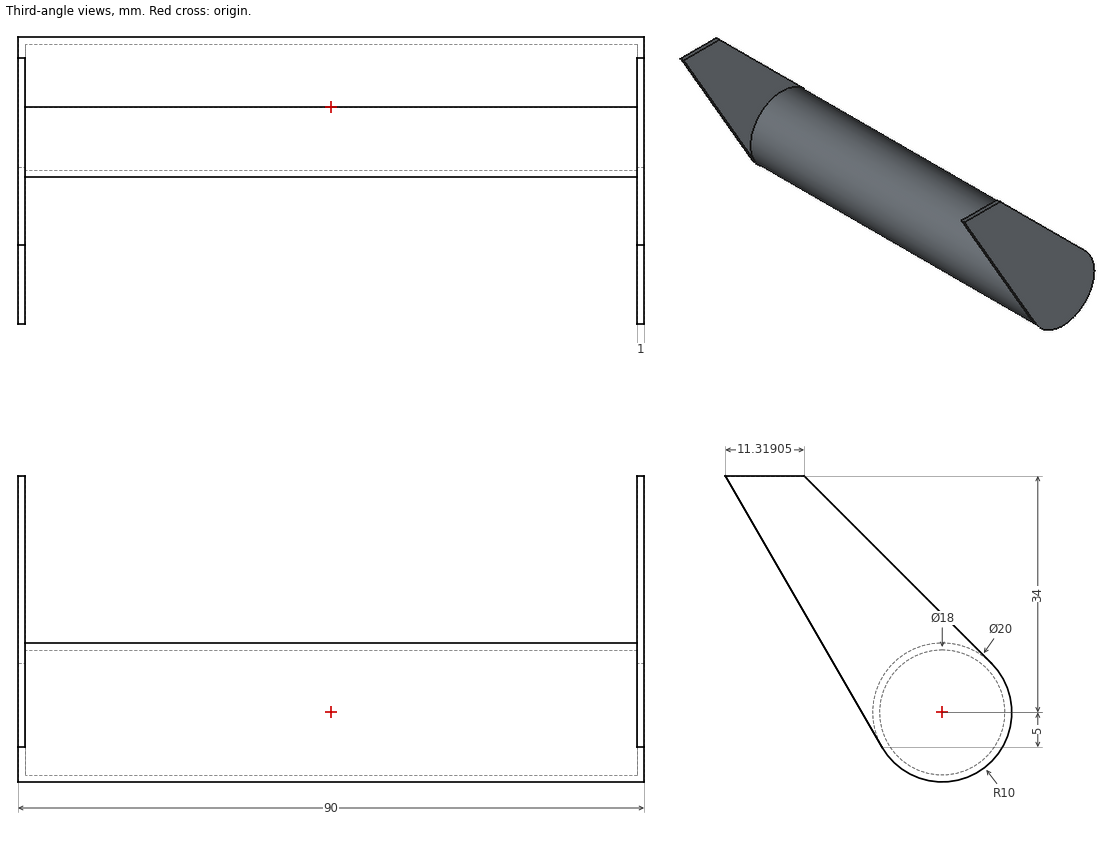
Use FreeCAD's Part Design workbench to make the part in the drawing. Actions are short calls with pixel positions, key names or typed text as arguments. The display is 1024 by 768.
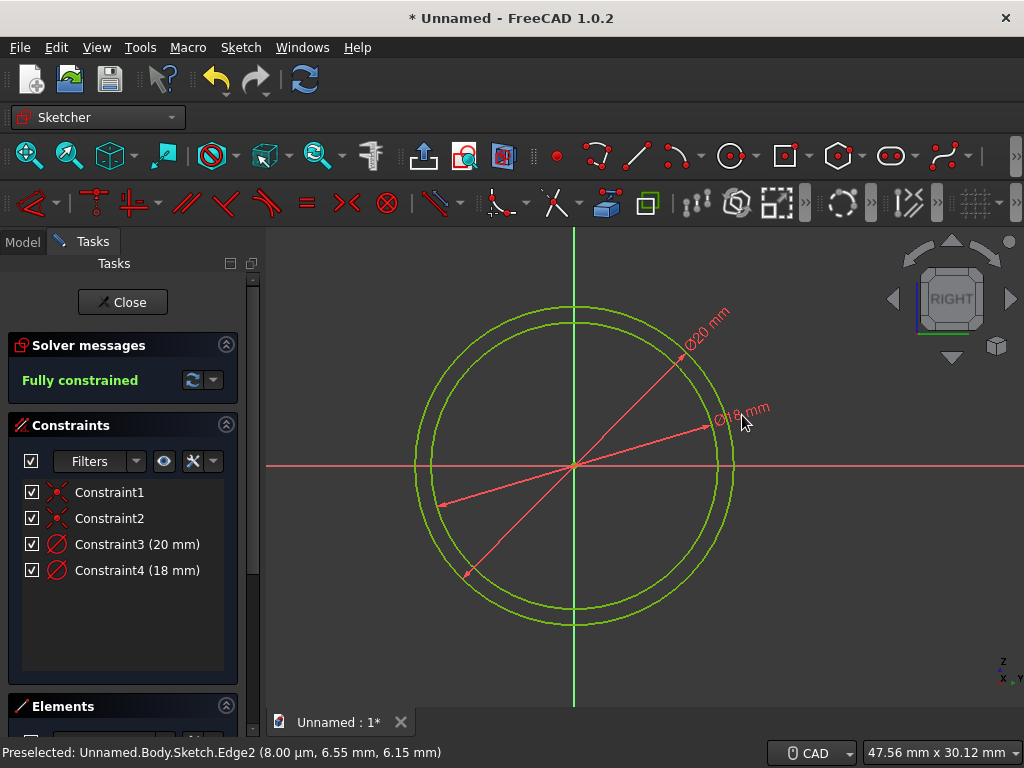
click(123, 302)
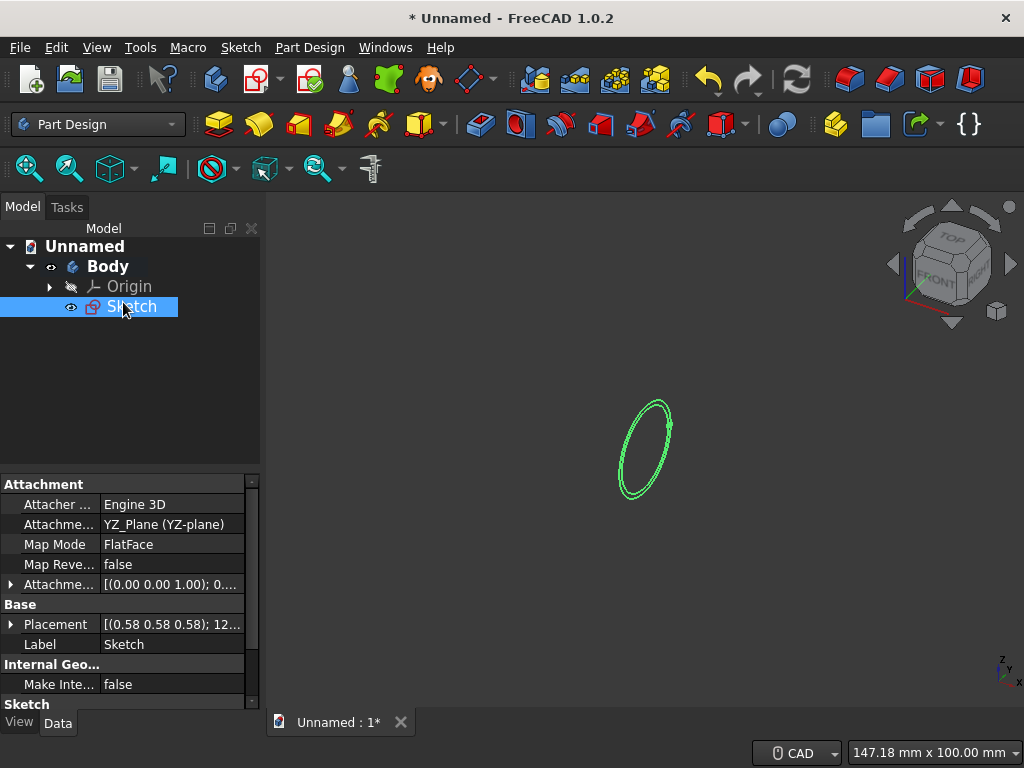
click(220, 124)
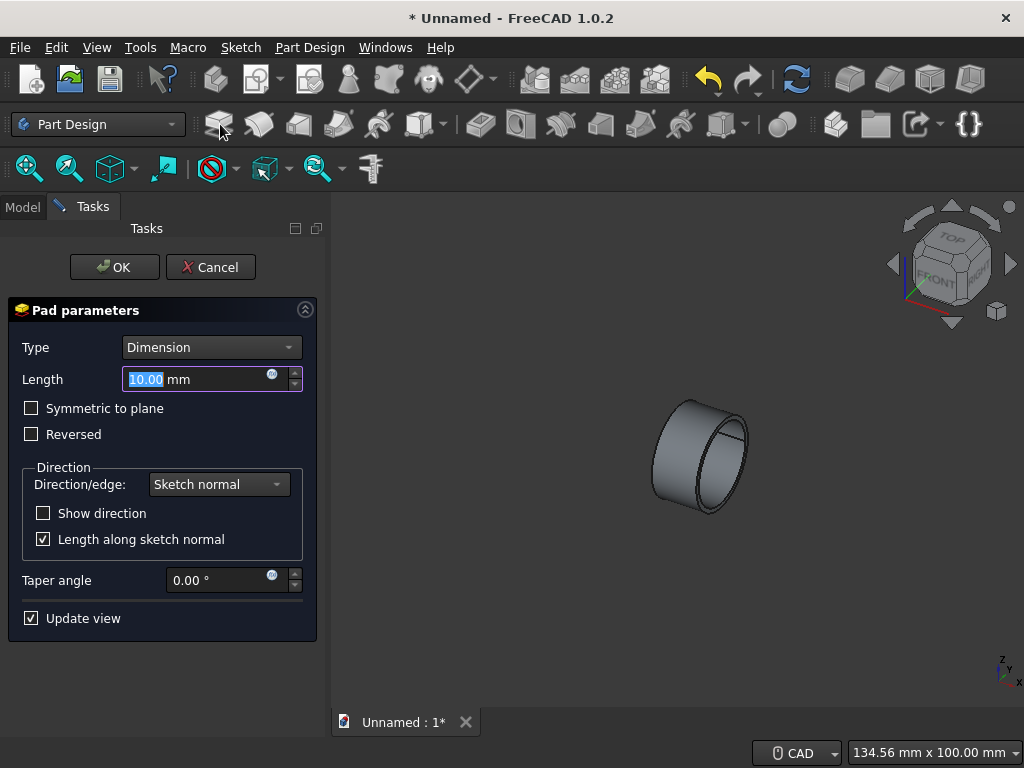
text(90)
key(Tab)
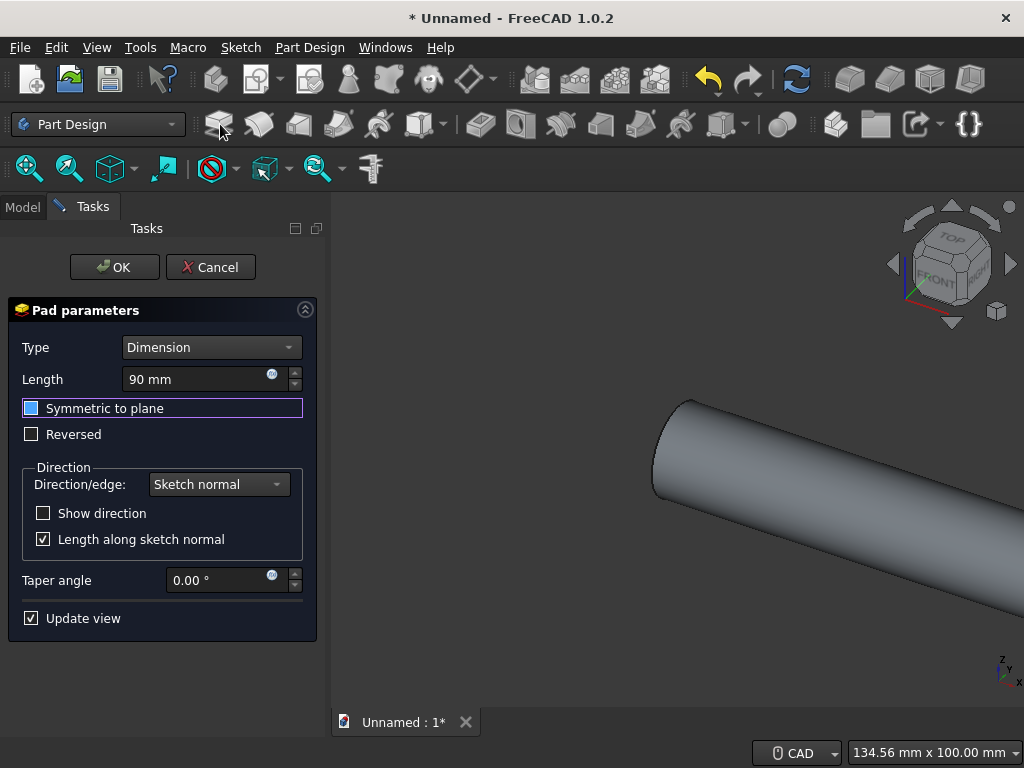
click(30, 408)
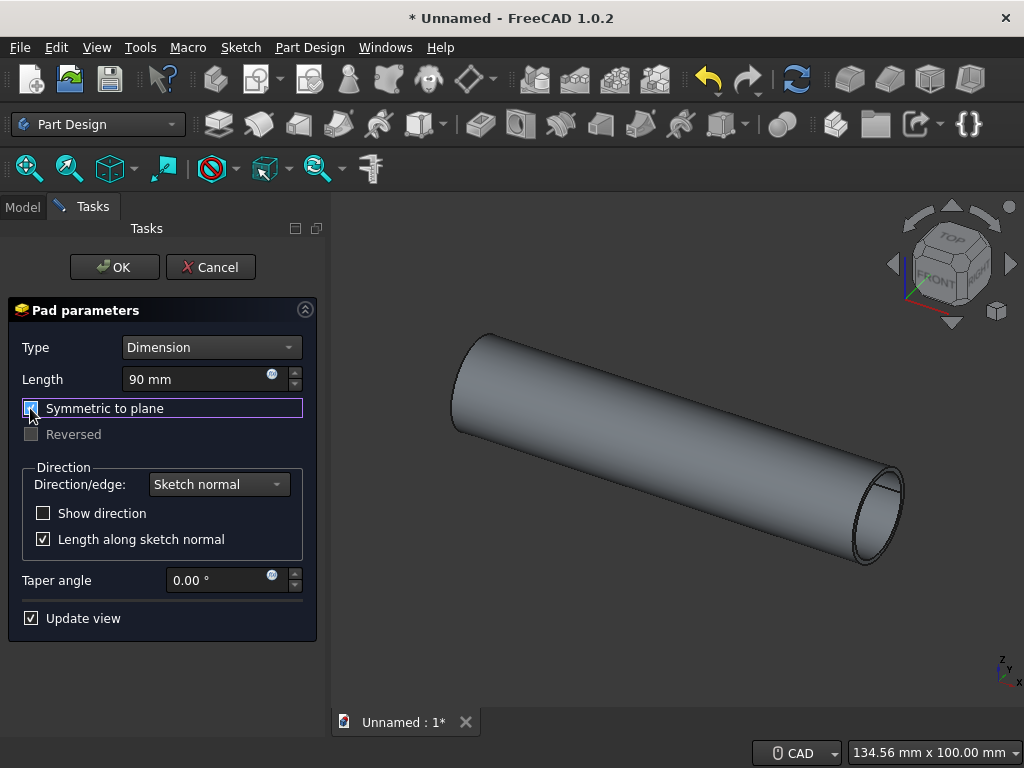
click(115, 267)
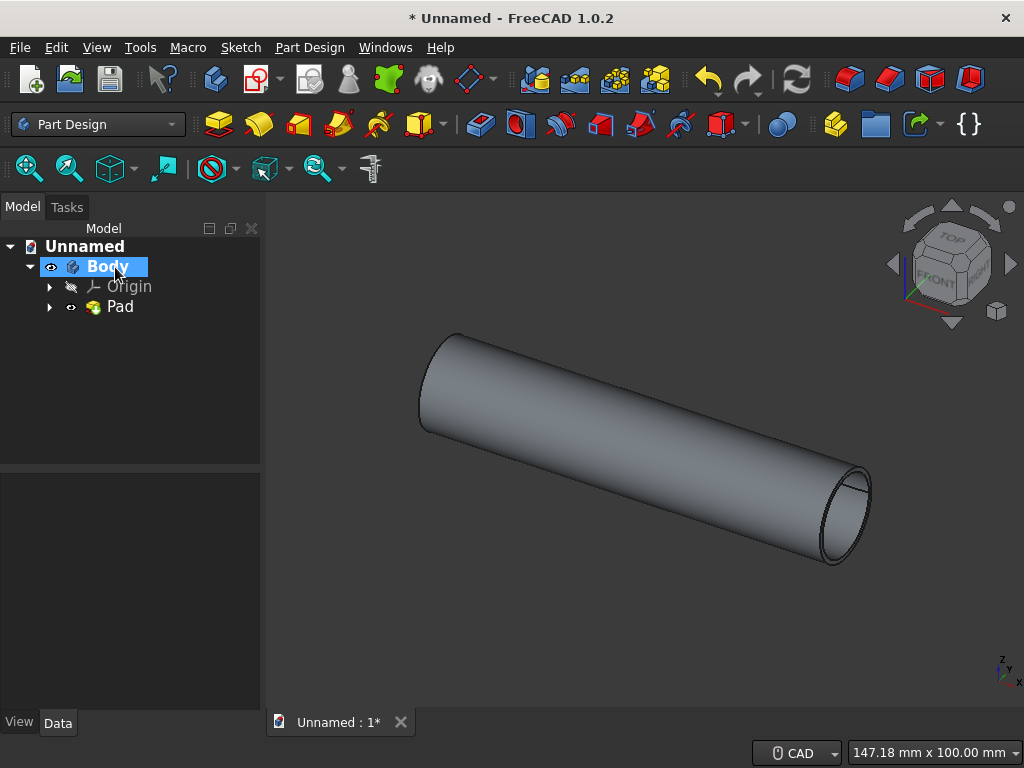
scroll(824, 525, up, 15)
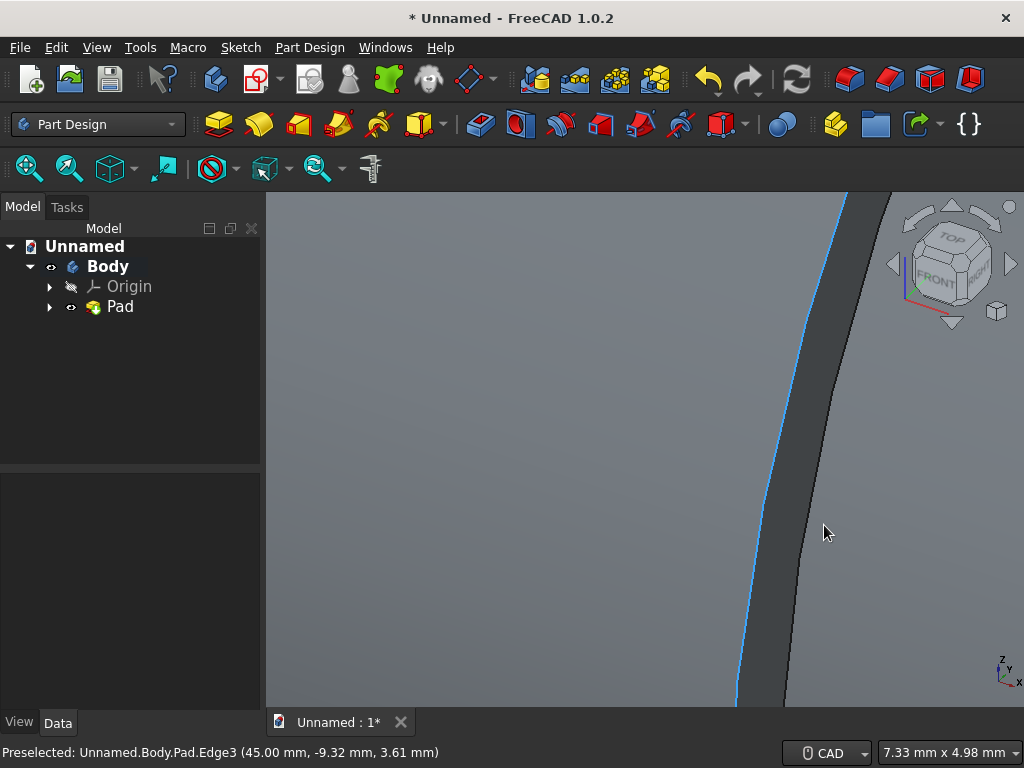
scroll(803, 528, up, 6)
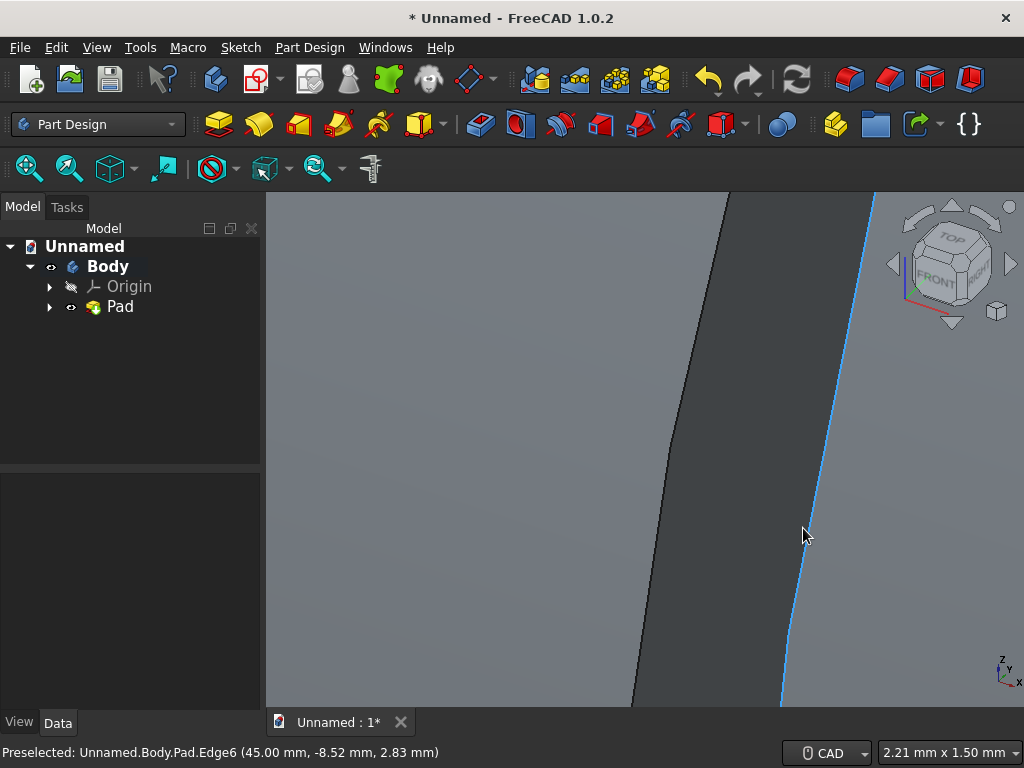
click(800, 530)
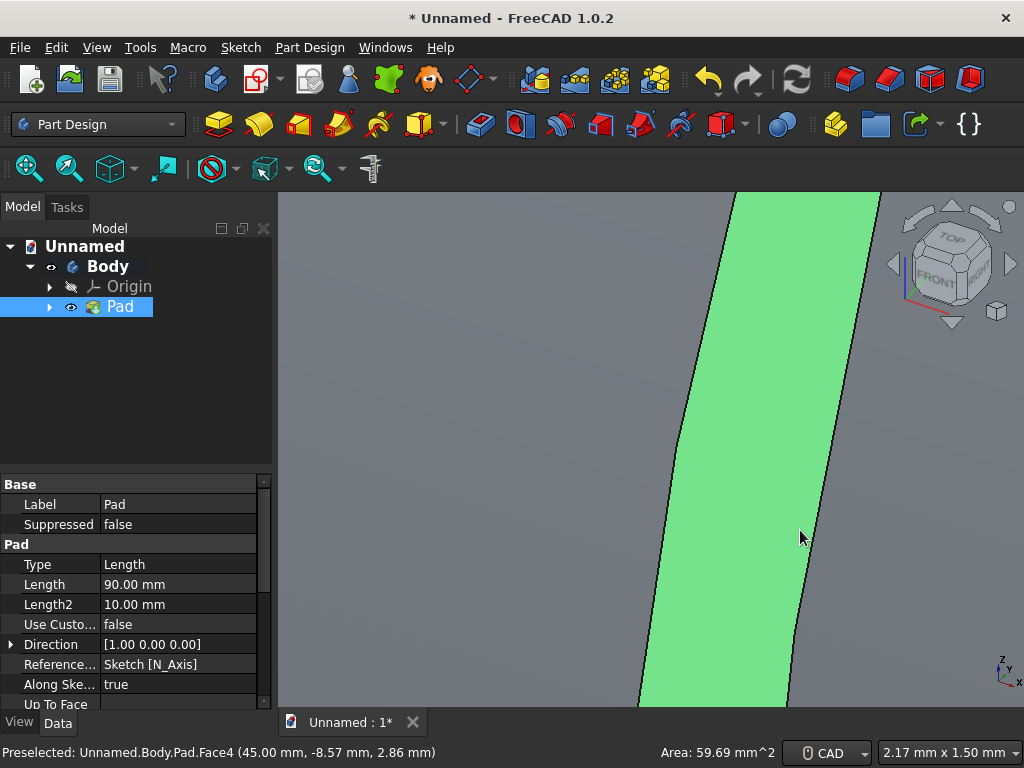
click(256, 80)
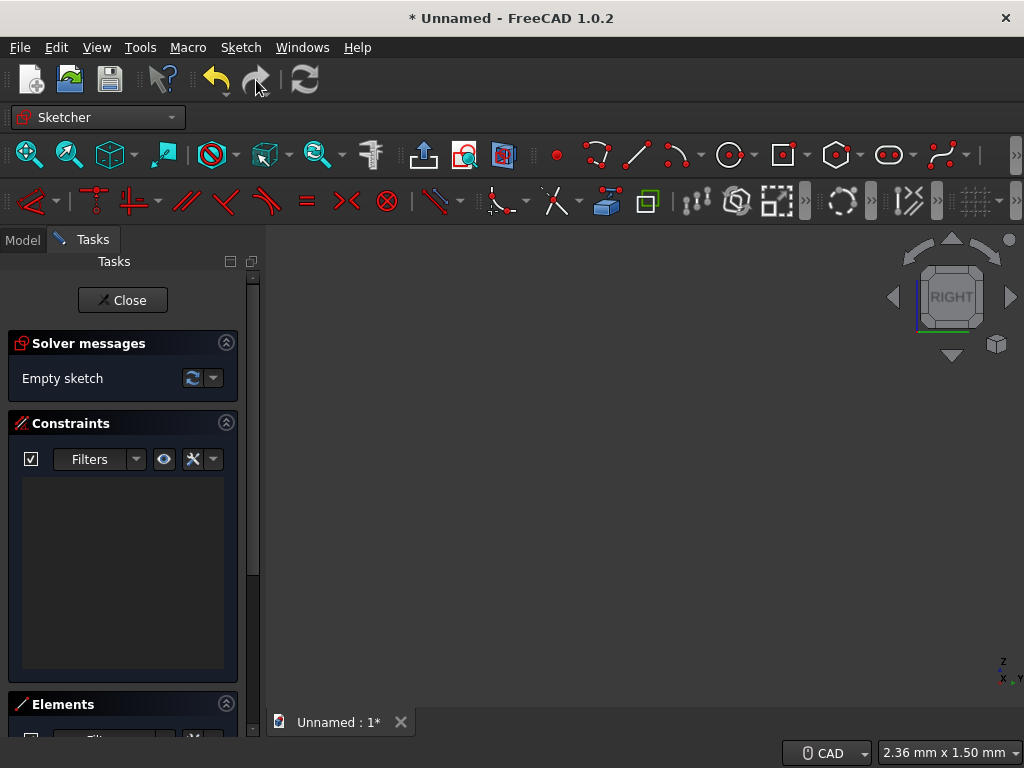
scroll(576, 466, down, 15)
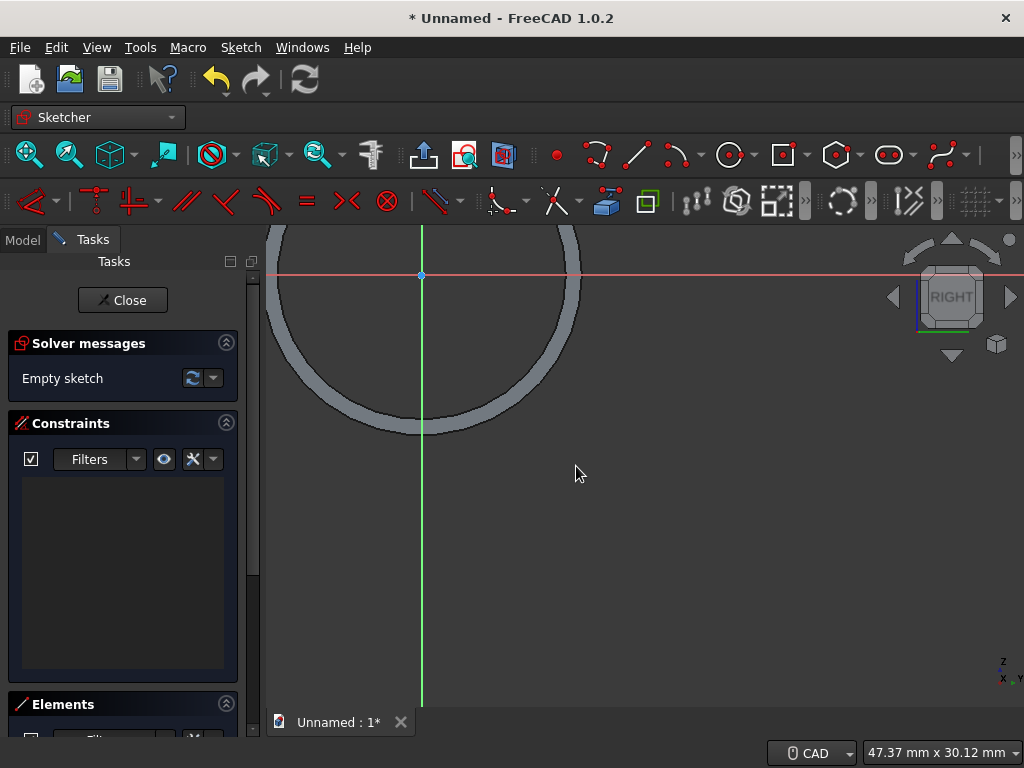
scroll(779, 679, down, 5)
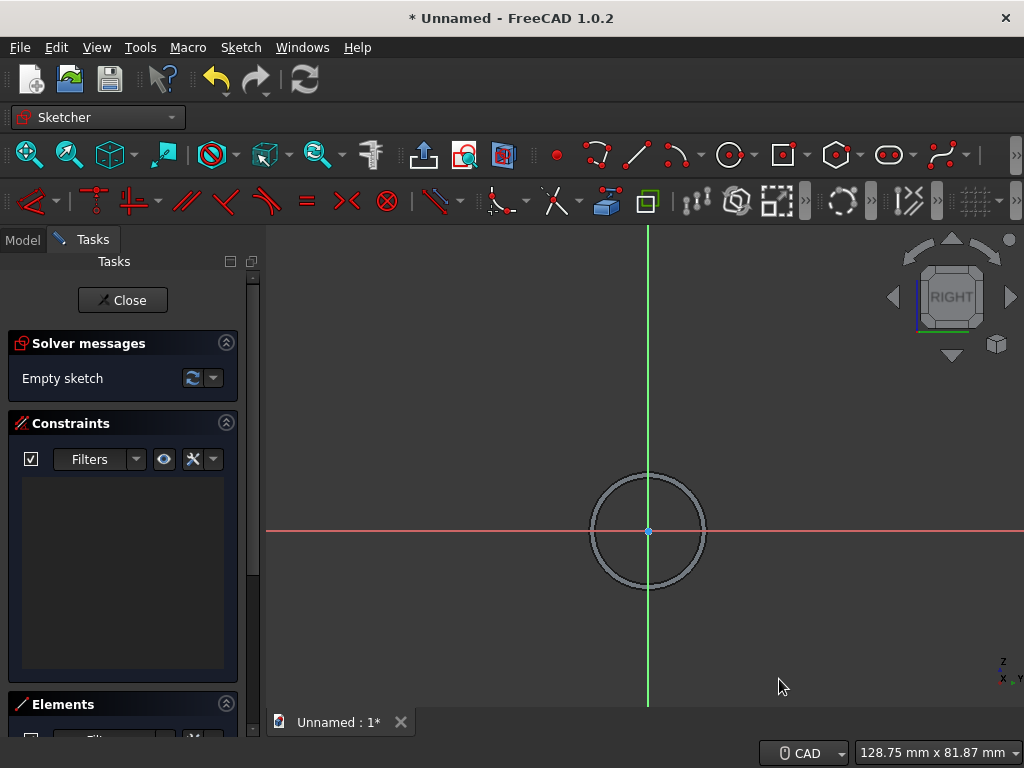
click(598, 156)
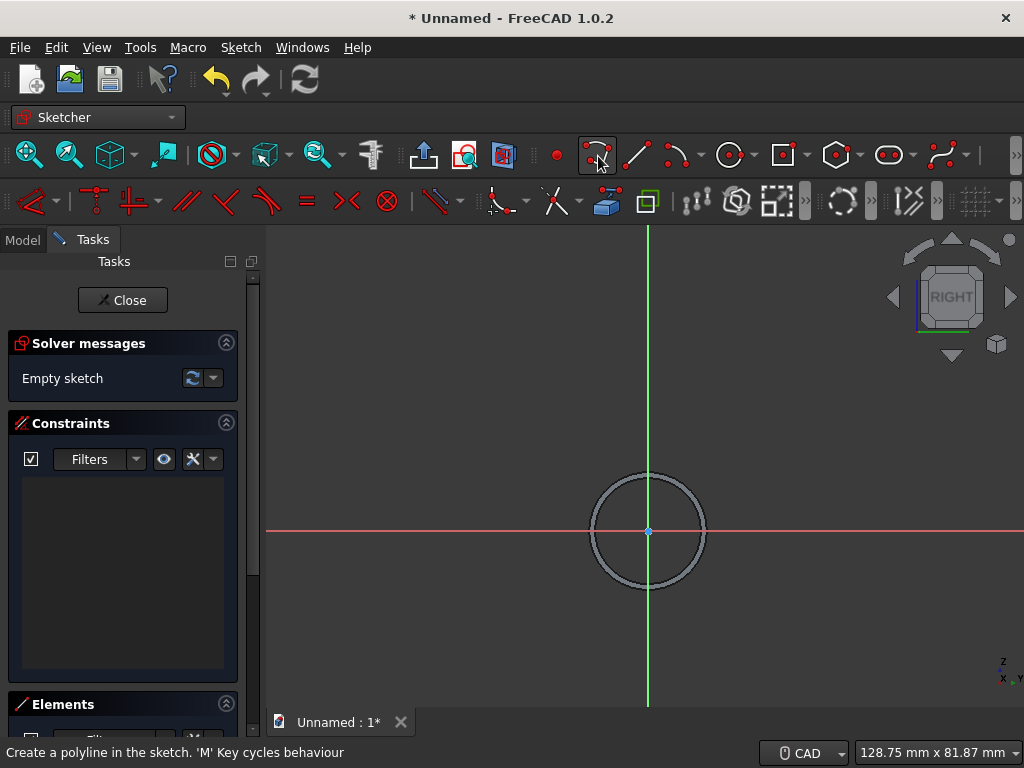
click(690, 489)
click(531, 331)
click(464, 331)
click(597, 561)
right_click(597, 561)